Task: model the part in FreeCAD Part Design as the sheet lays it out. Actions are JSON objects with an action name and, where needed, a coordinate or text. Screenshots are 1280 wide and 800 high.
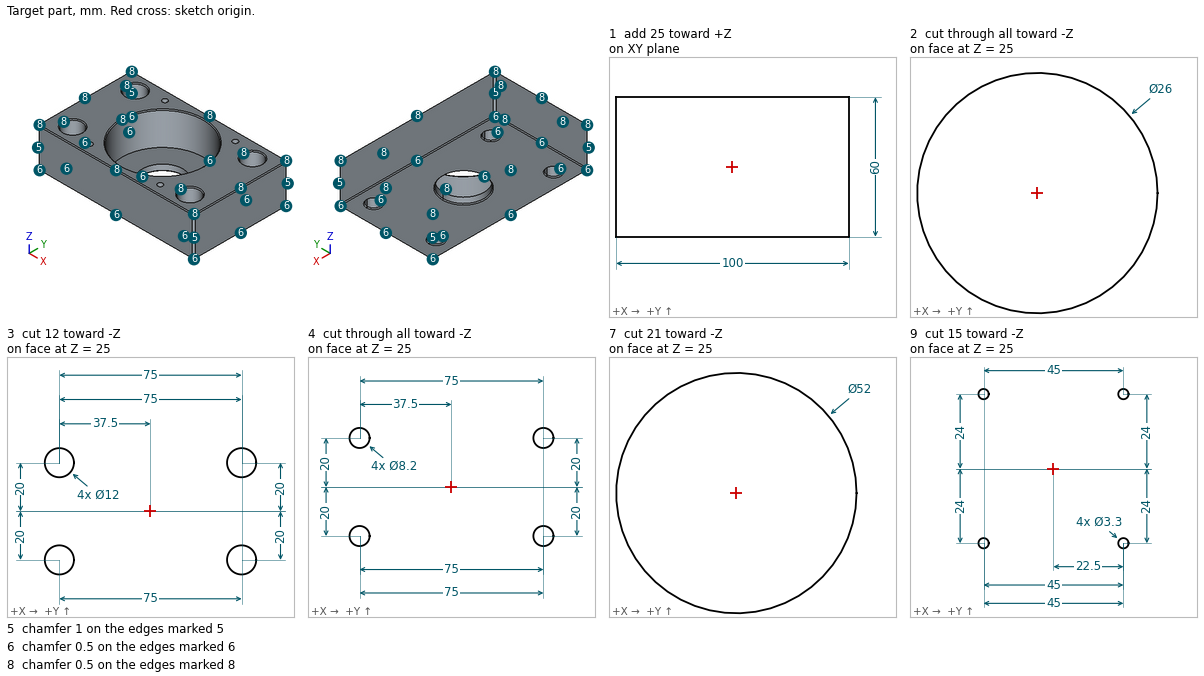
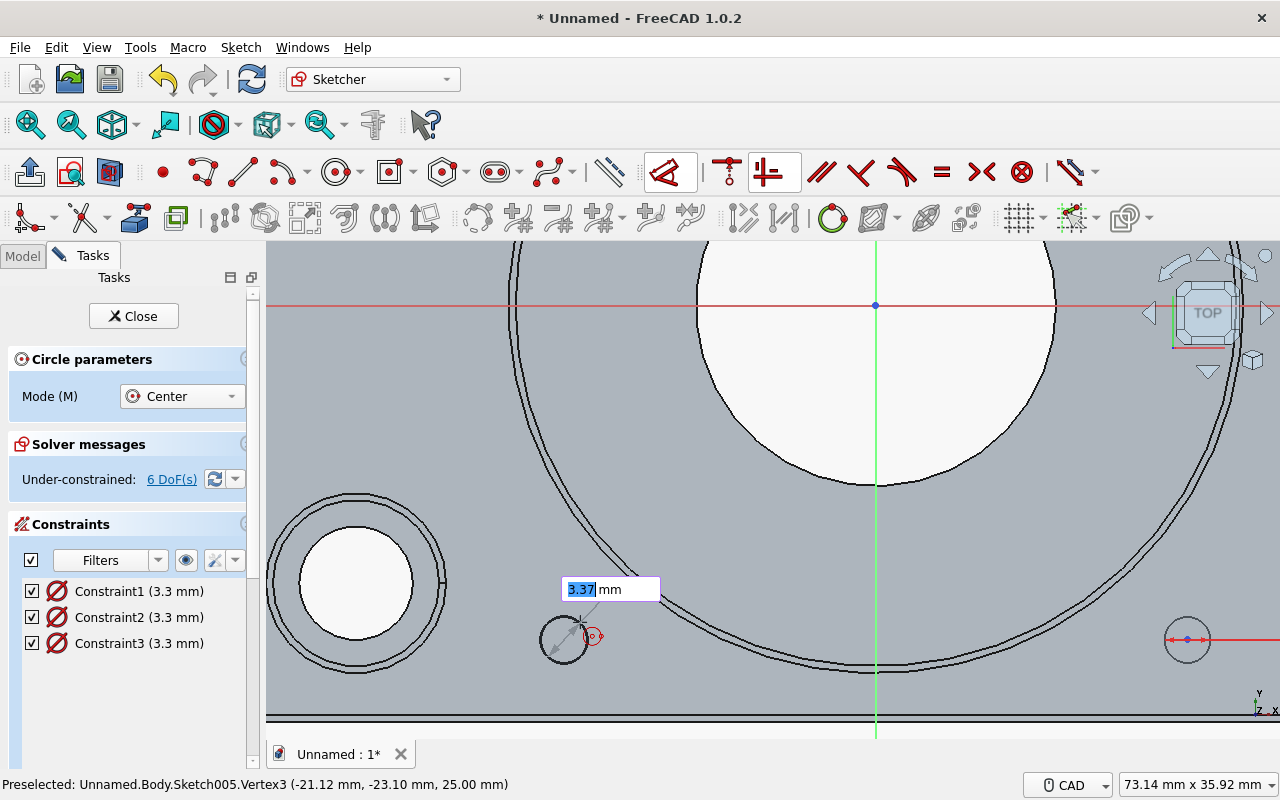
{"action": "type", "text": "3.3"}
{"action": "key", "text": "Return"}
{"action": "key", "text": "Escape"}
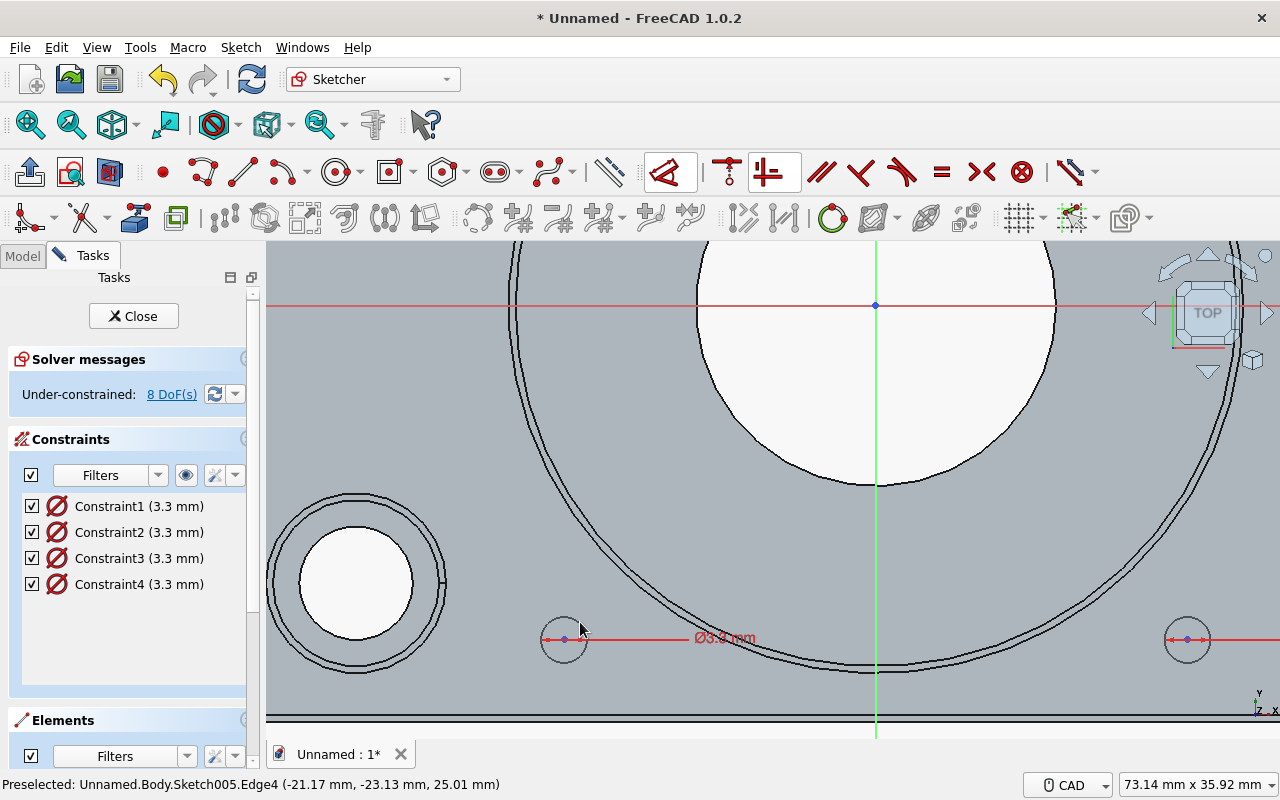
{"action": "scroll", "coordinate": [565, 640], "scroll_direction": "down", "scroll_amount": 4}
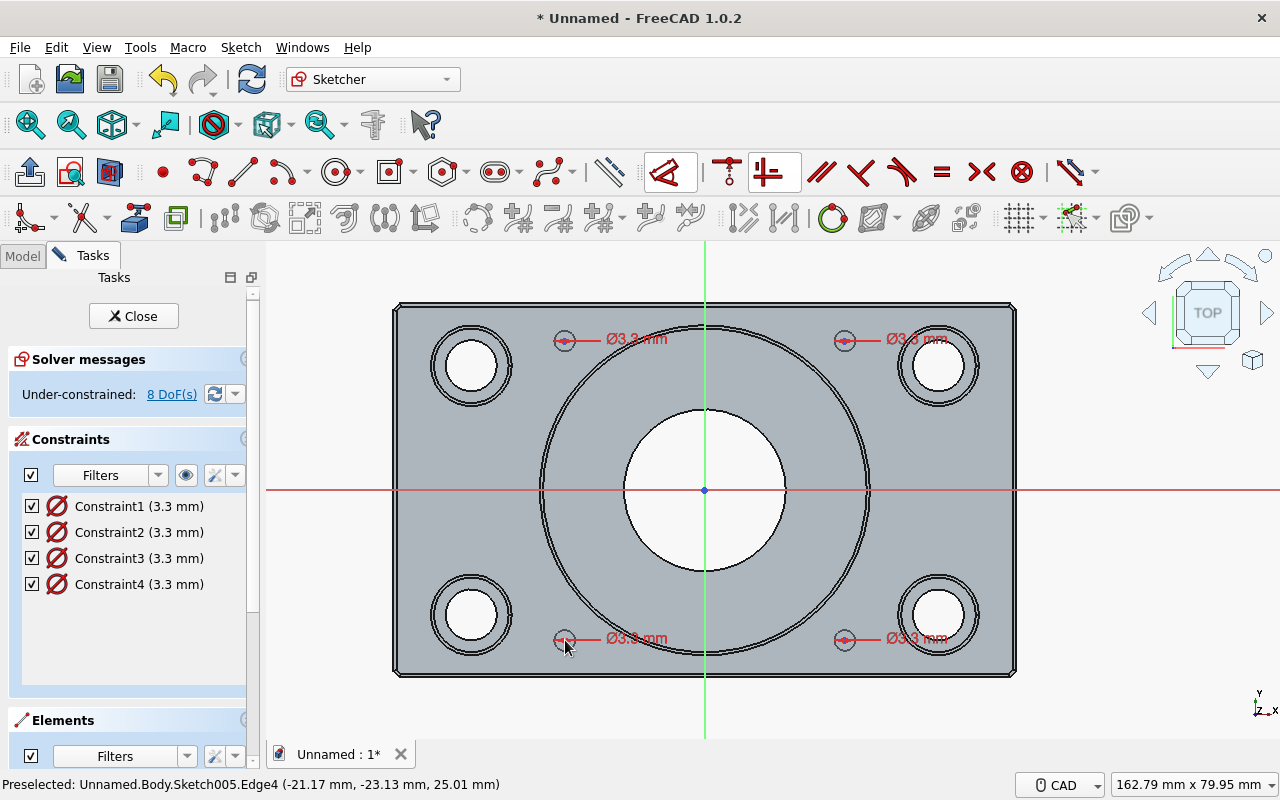
{"action": "left_click", "coordinate": [845, 640]}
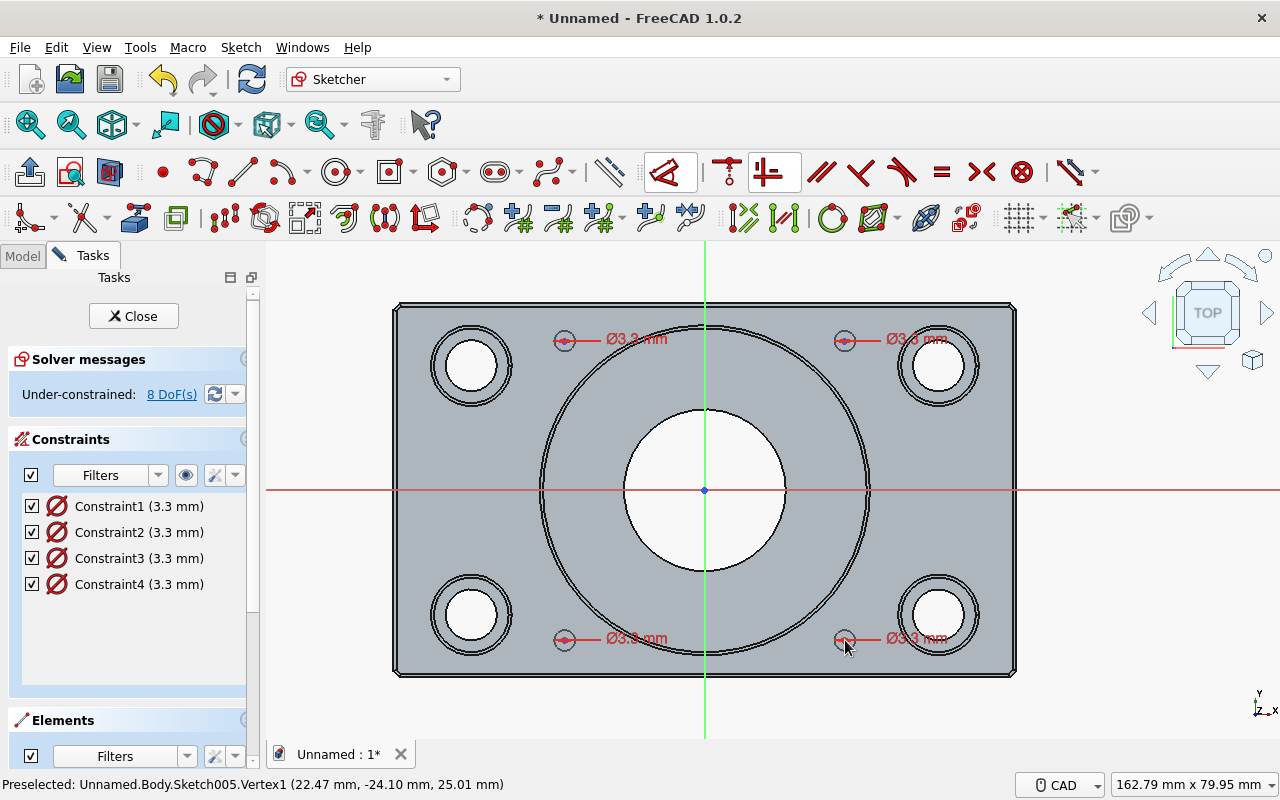
{"action": "key", "text": "i"}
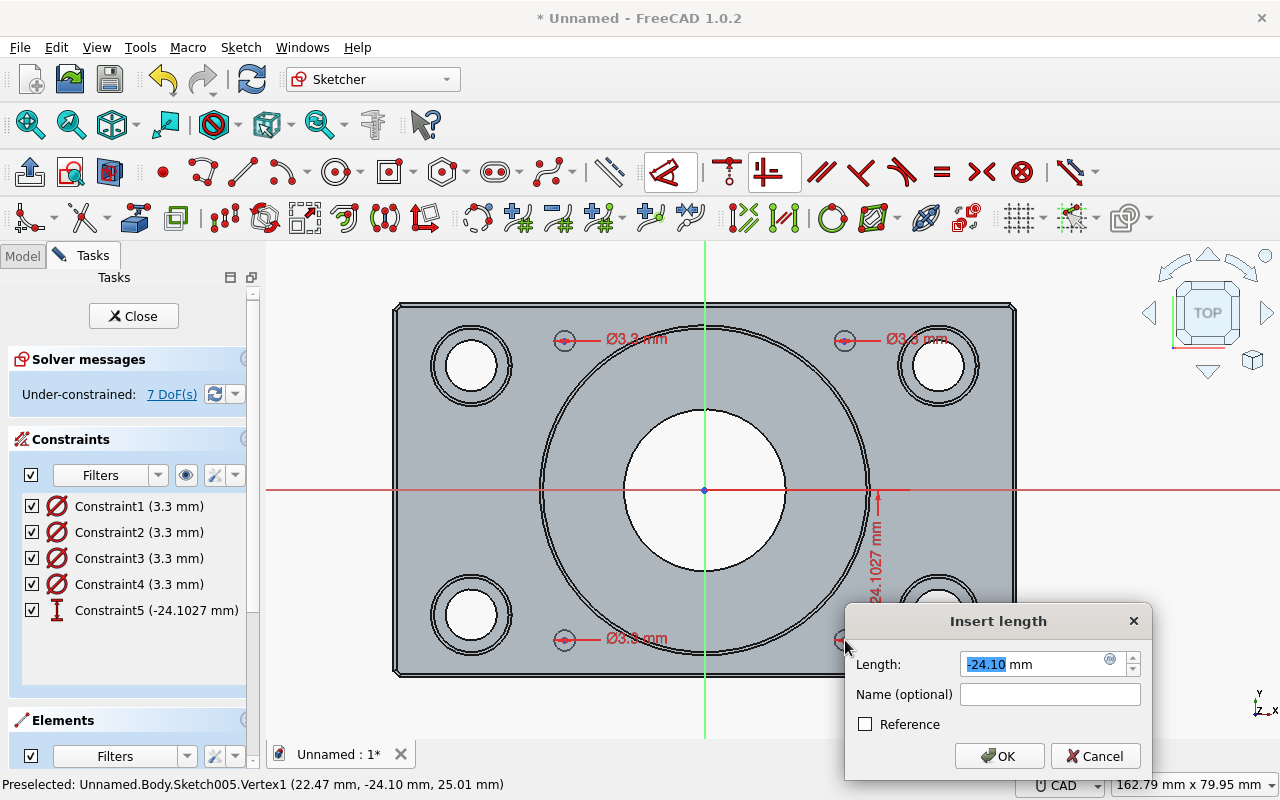
{"action": "type", "text": "-24"}
{"action": "key", "text": "Return"}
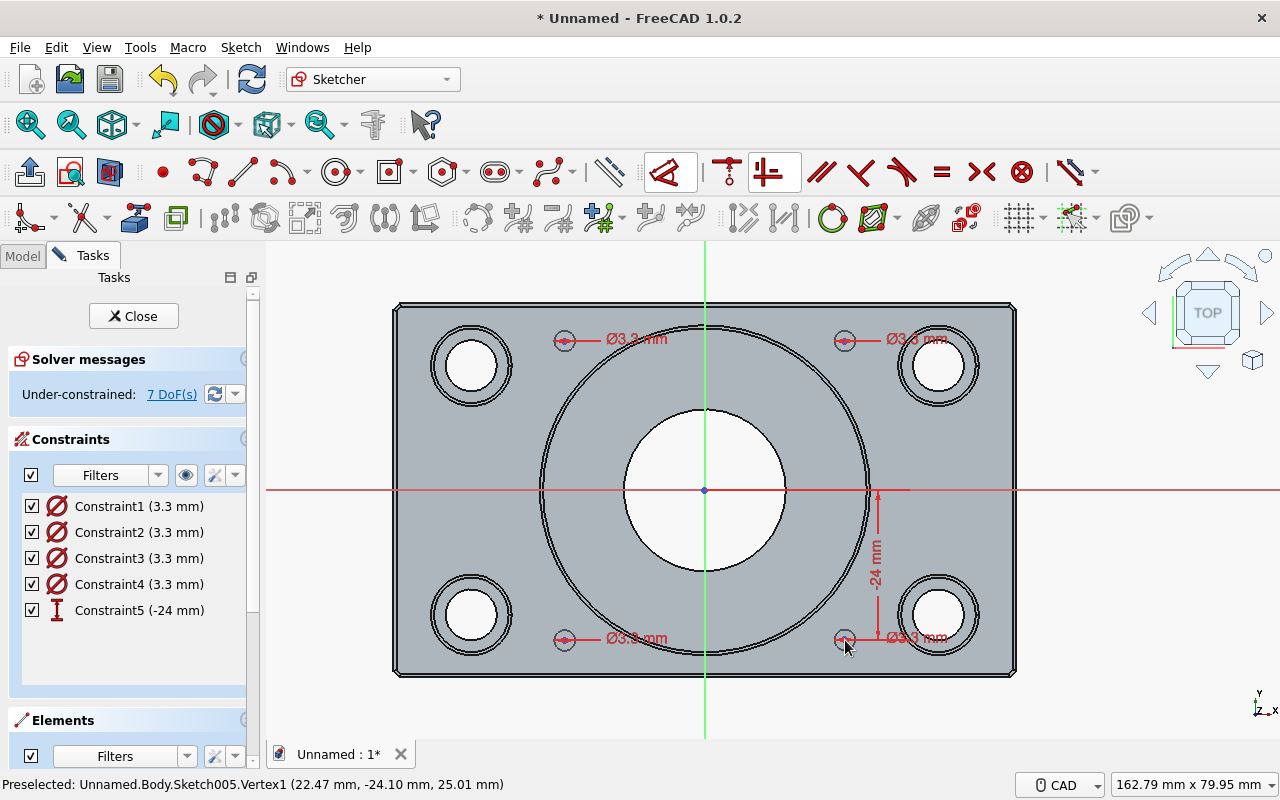
{"action": "left_click", "coordinate": [845, 341]}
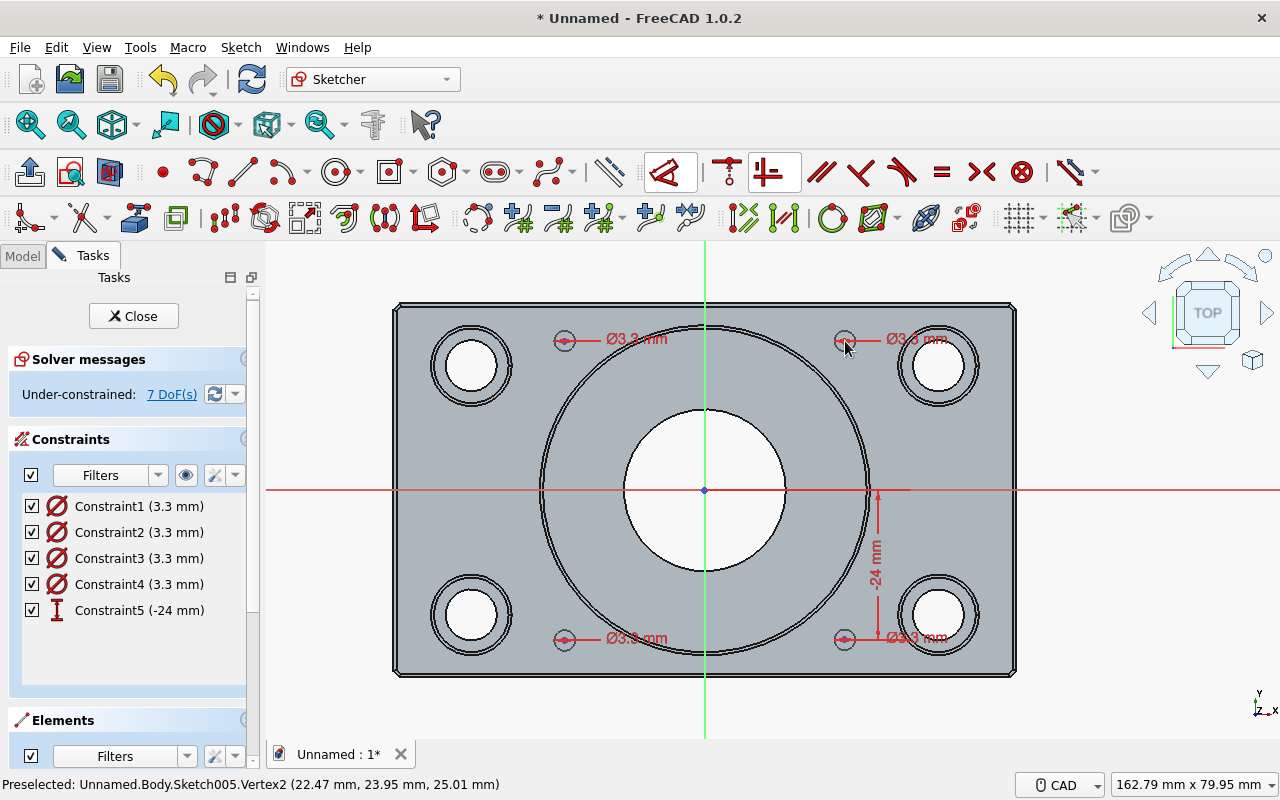
{"action": "left_click", "coordinate": [692, 172]}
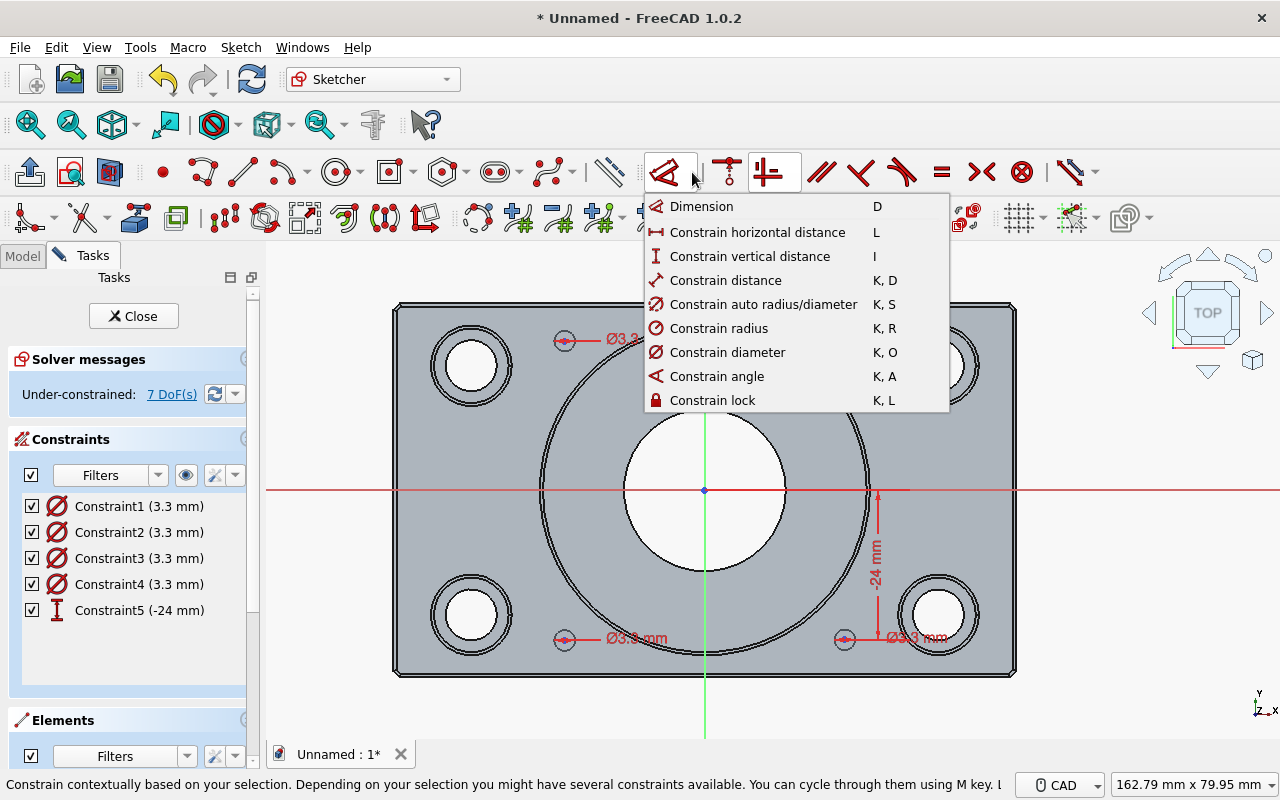
{"action": "left_click", "coordinate": [797, 256]}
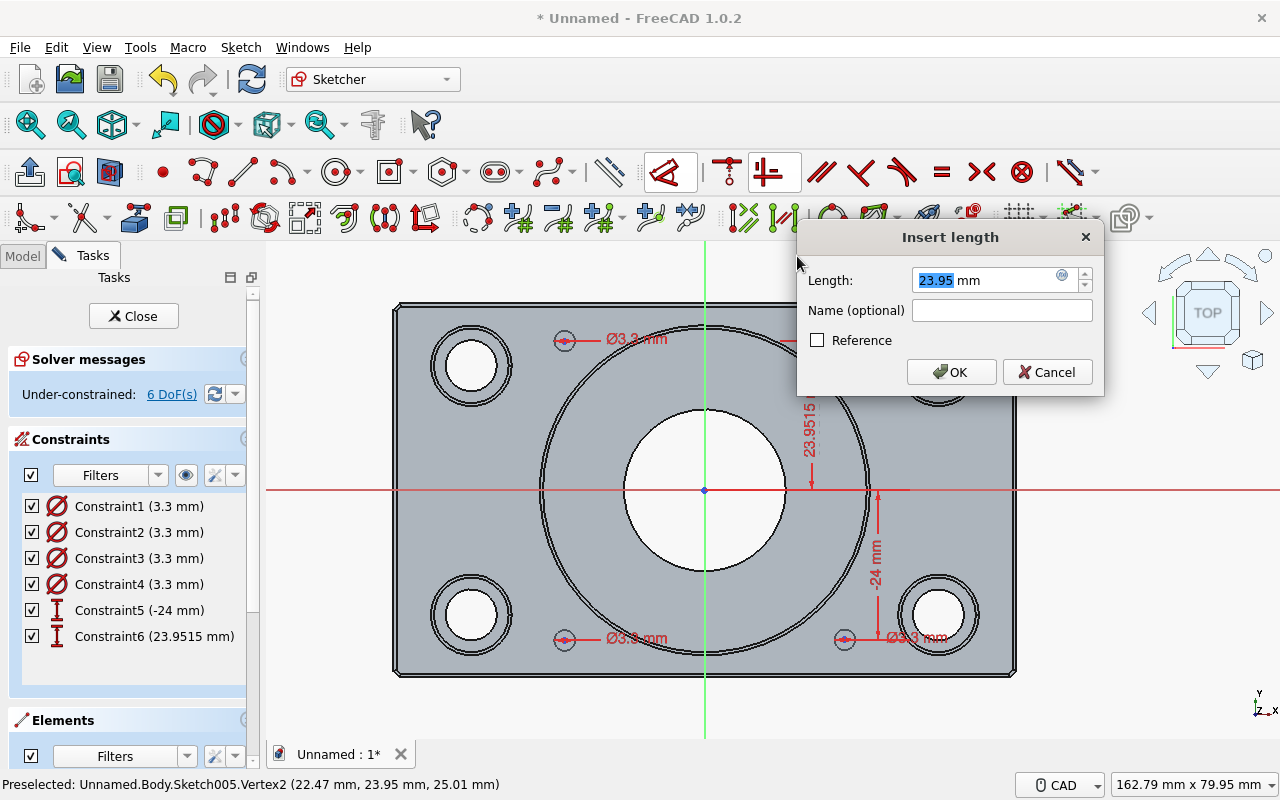
{"action": "type", "text": "24"}
{"action": "key", "text": "Return"}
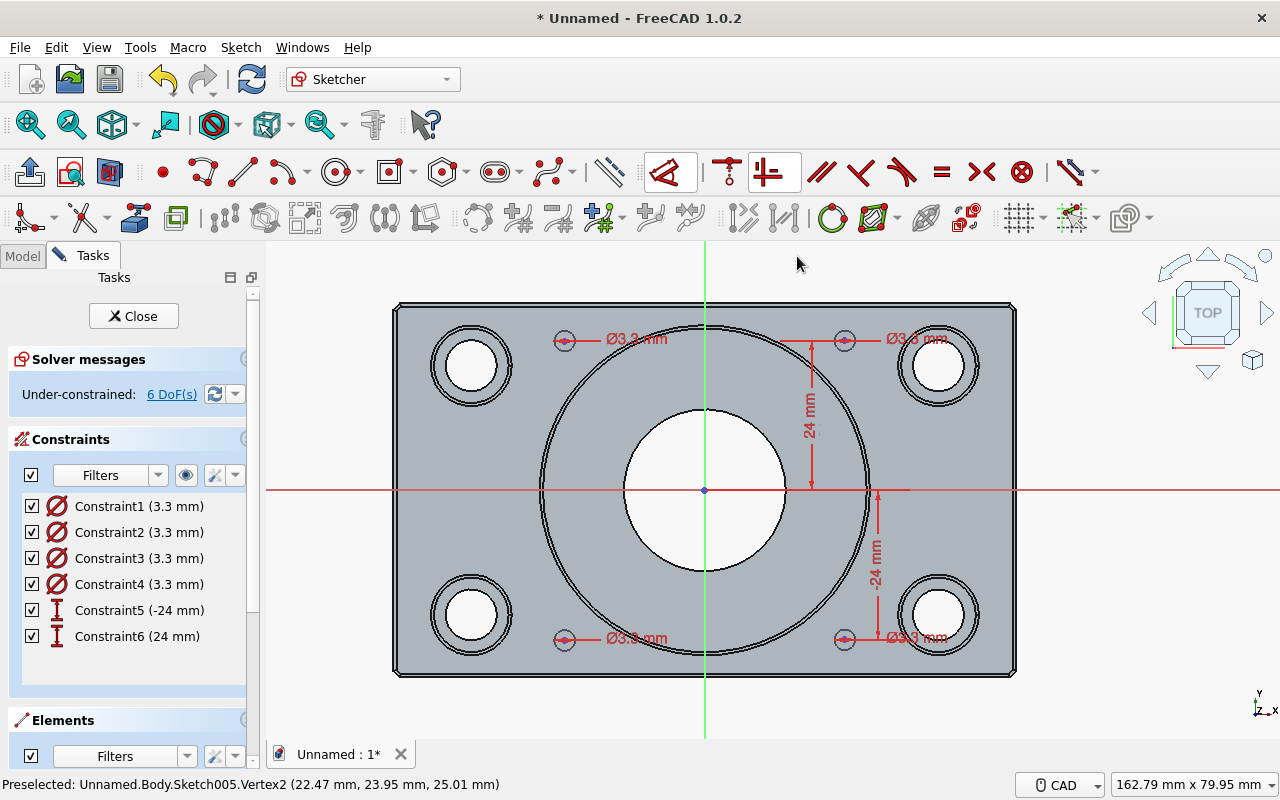
{"action": "left_click", "coordinate": [565, 341]}